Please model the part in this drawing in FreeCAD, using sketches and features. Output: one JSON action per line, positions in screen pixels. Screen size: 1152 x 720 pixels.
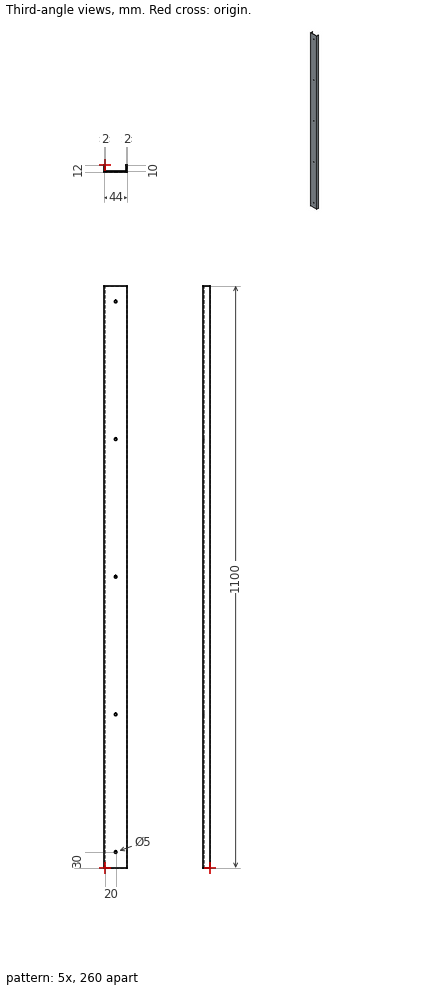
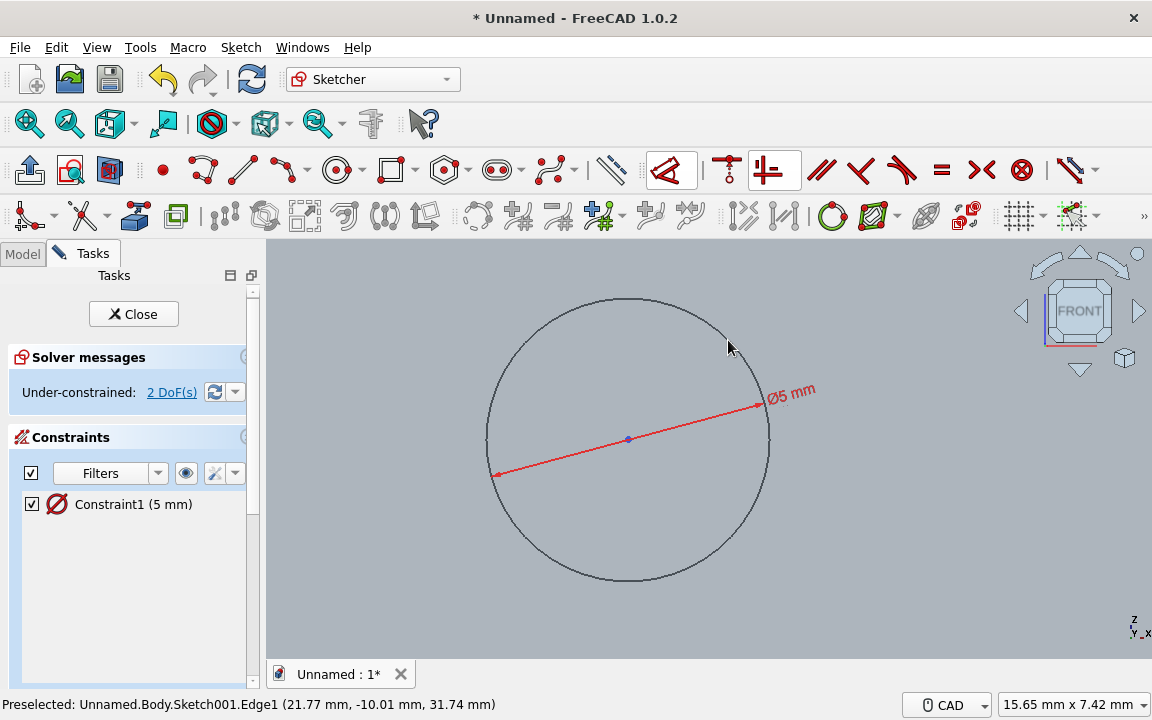
{"action": "left_click", "coordinate": [628, 440]}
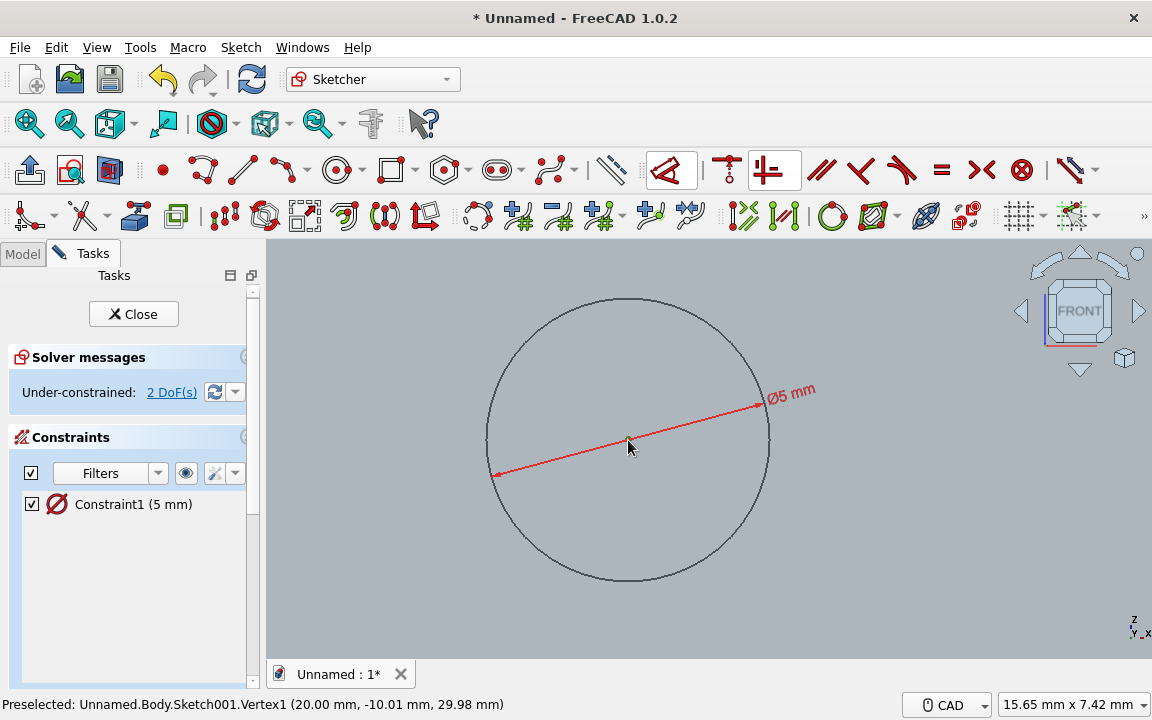
{"action": "key", "text": "l"}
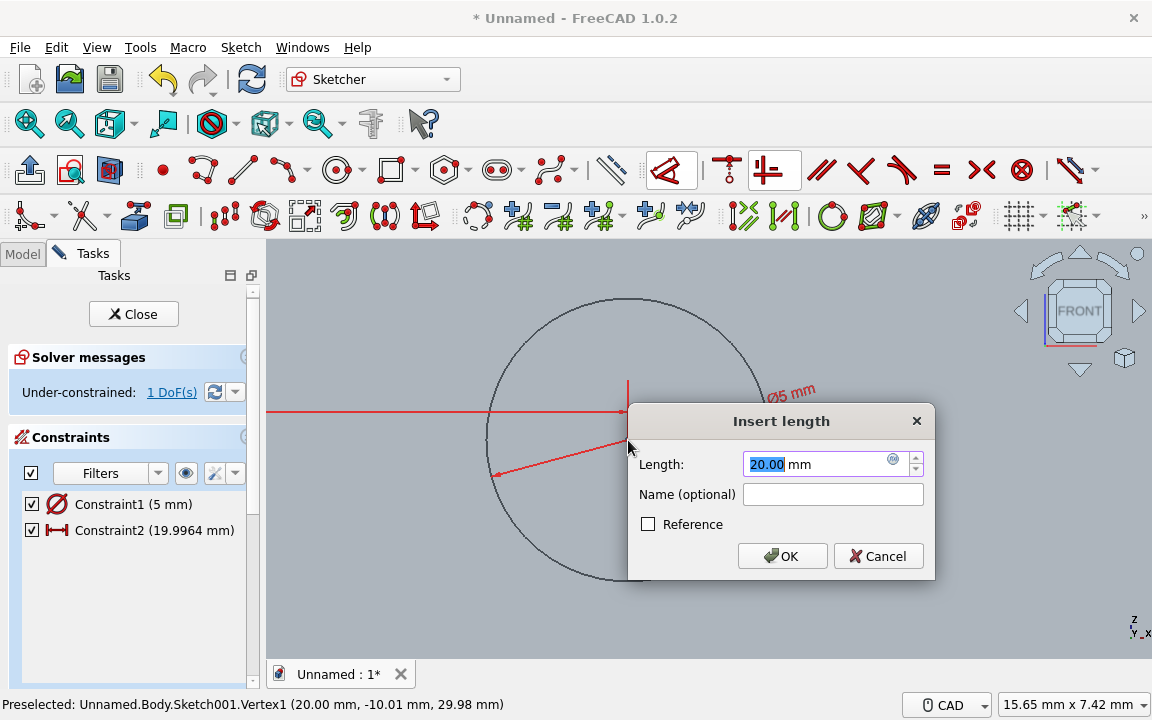
{"action": "type", "text": "20"}
{"action": "key", "text": "Return"}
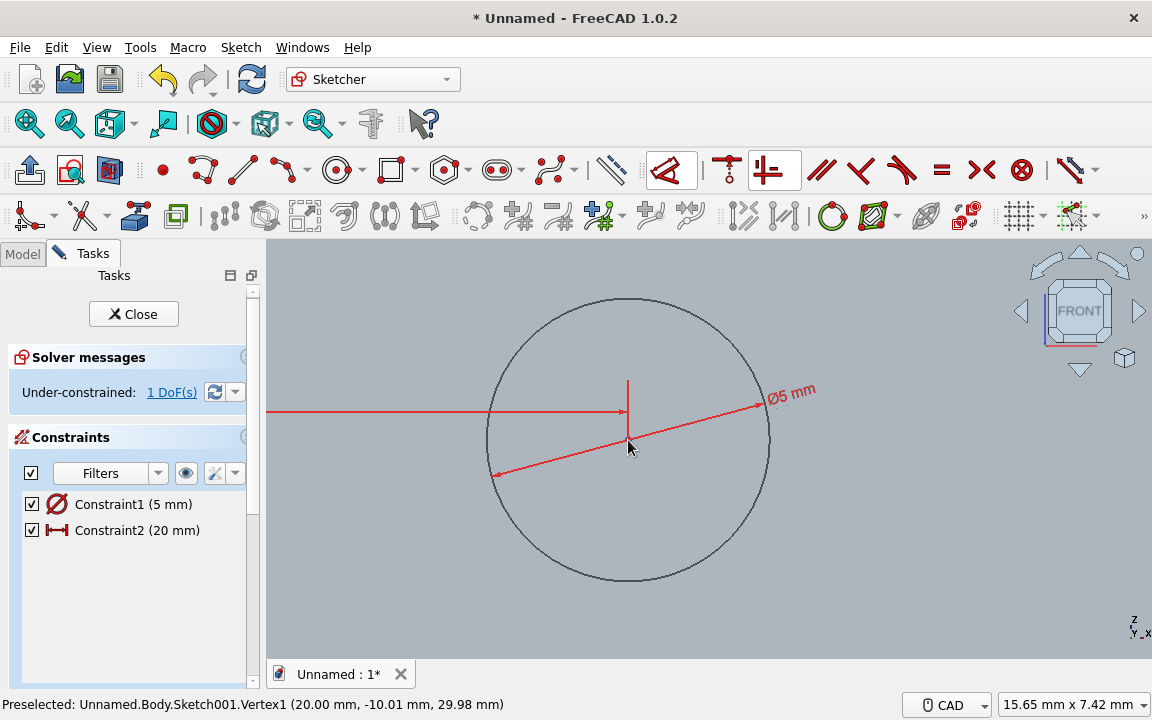
{"action": "left_click", "coordinate": [628, 440]}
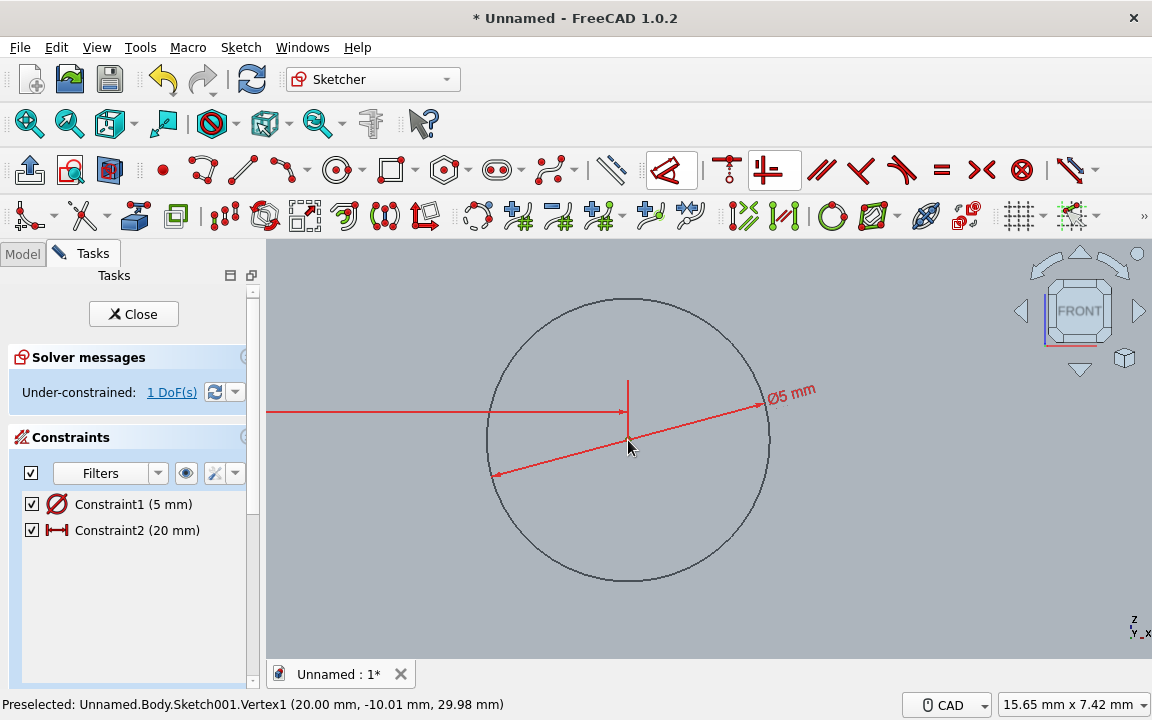
{"action": "left_click", "coordinate": [692, 170]}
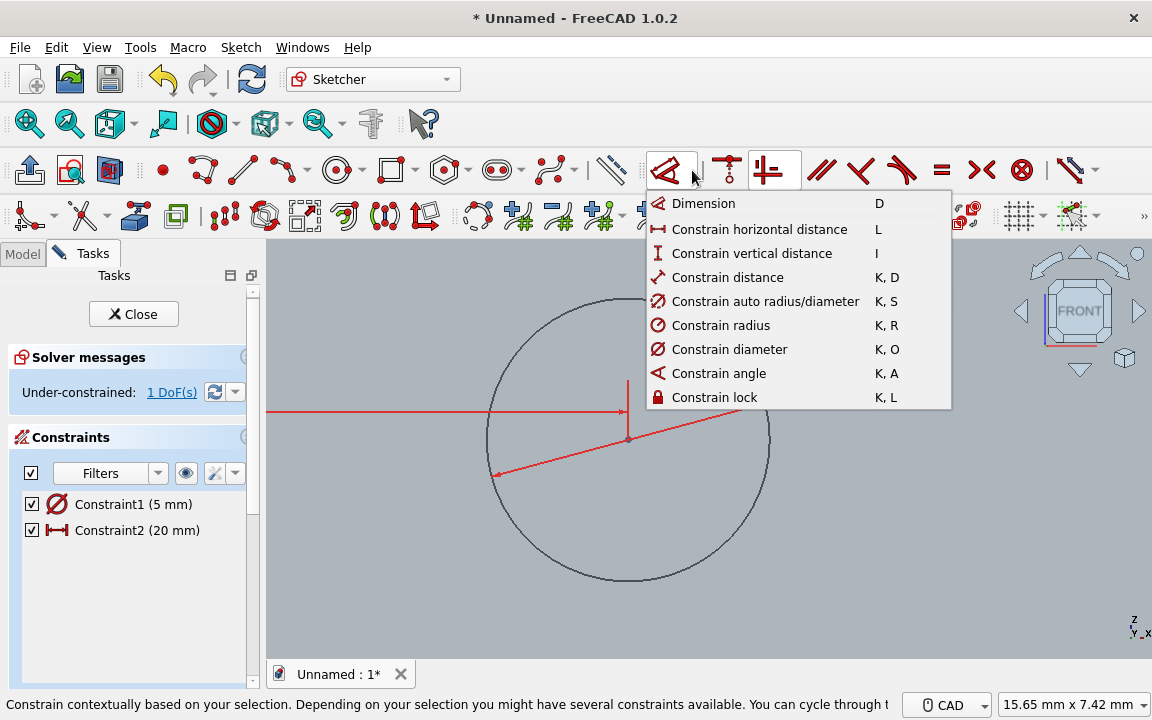
{"action": "left_click", "coordinate": [799, 253]}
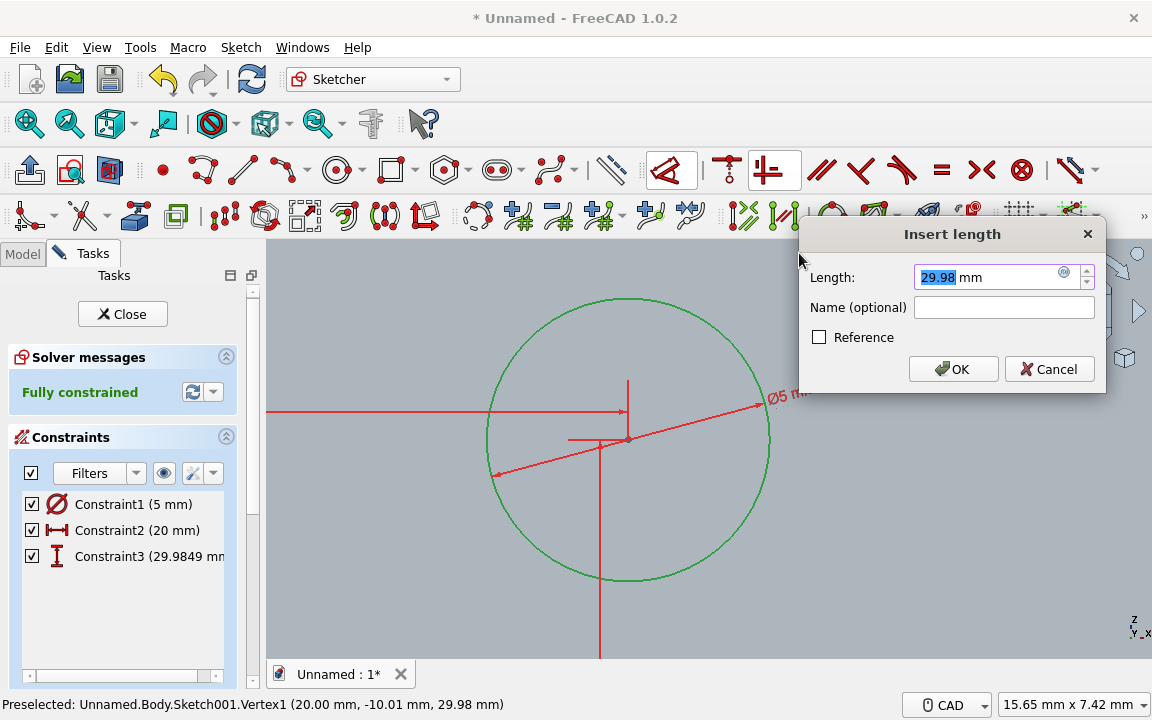
{"action": "type", "text": "30"}
{"action": "key", "text": "Return"}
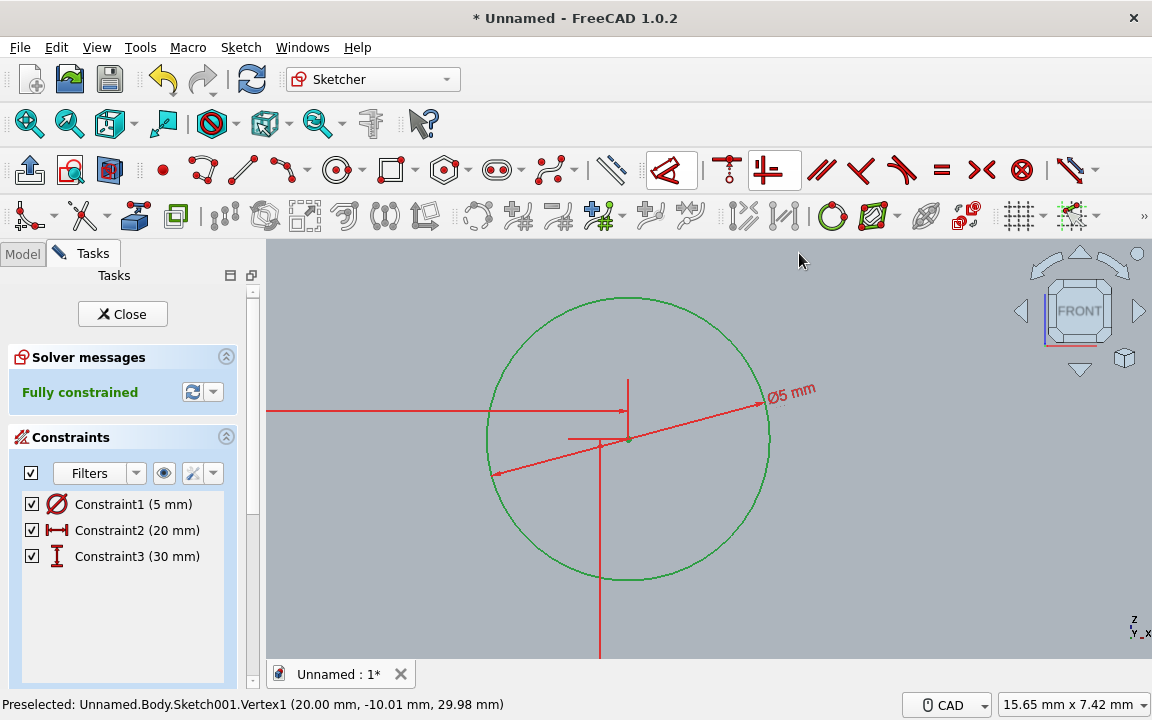
{"action": "left_click", "coordinate": [123, 314]}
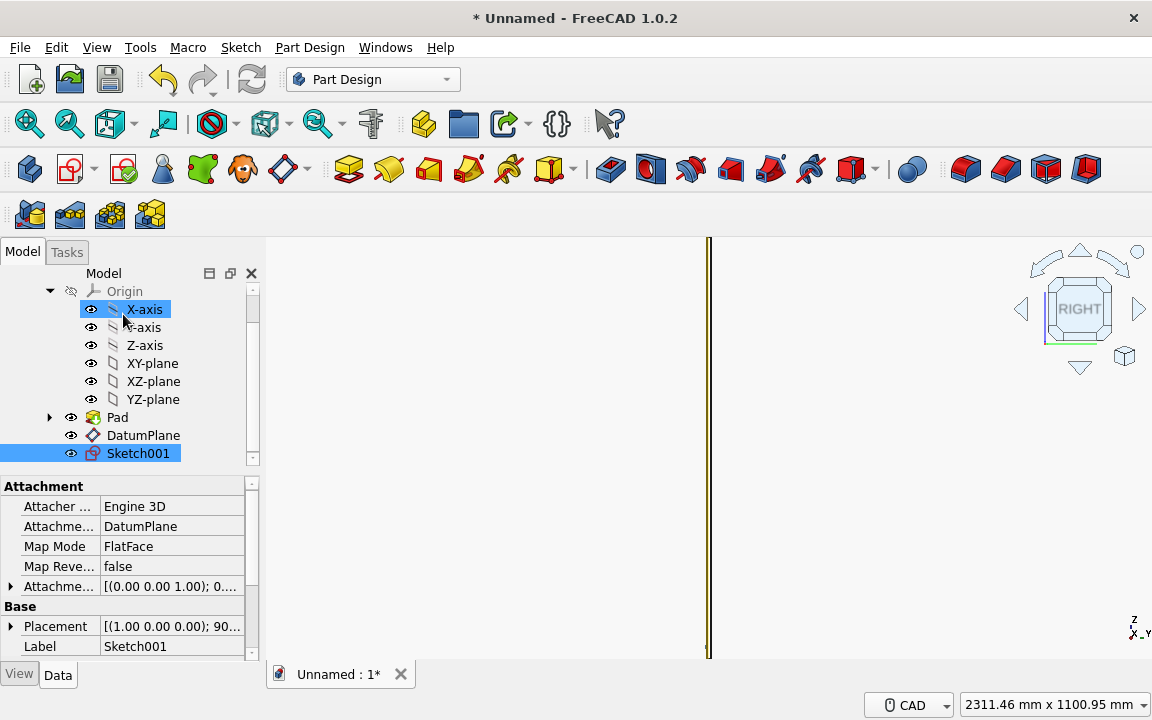
{"action": "left_click", "coordinate": [612, 170]}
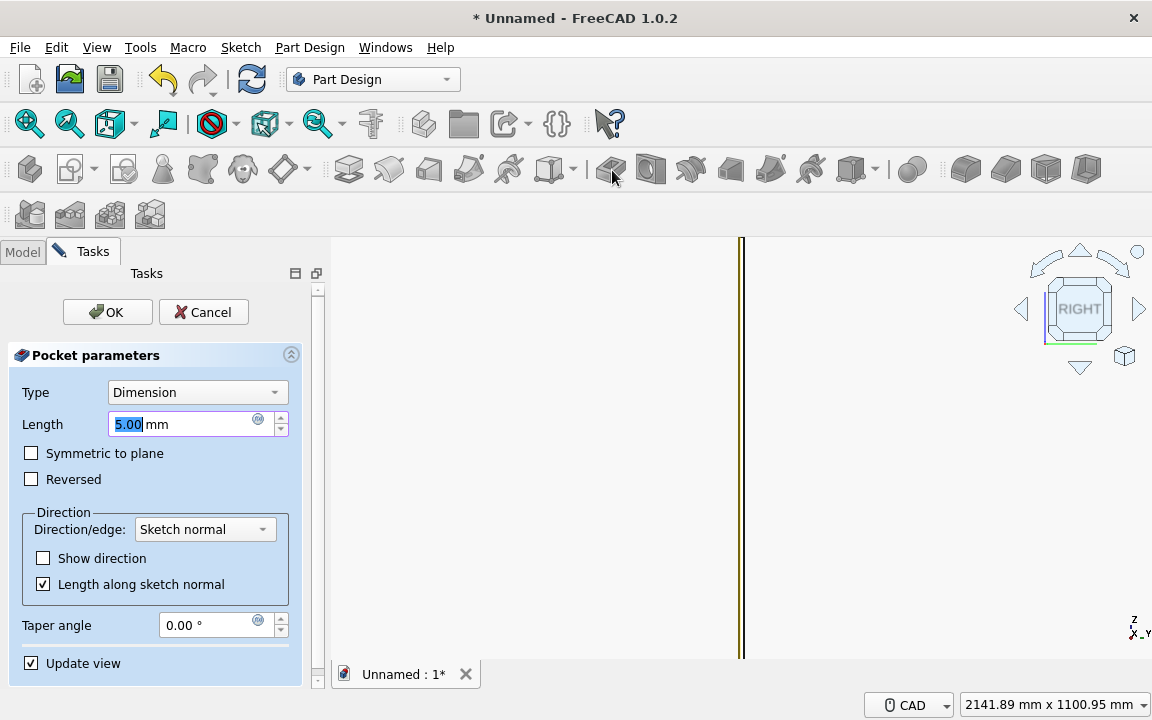
{"action": "left_click", "coordinate": [198, 392]}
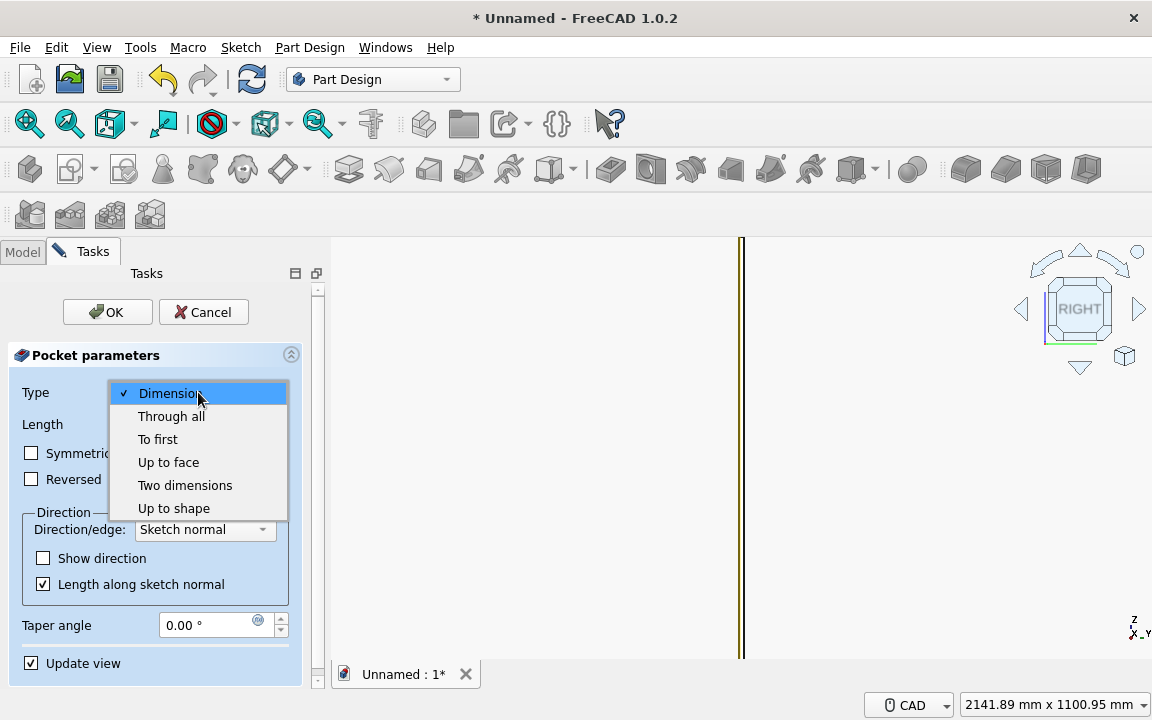
{"action": "left_click", "coordinate": [198, 416]}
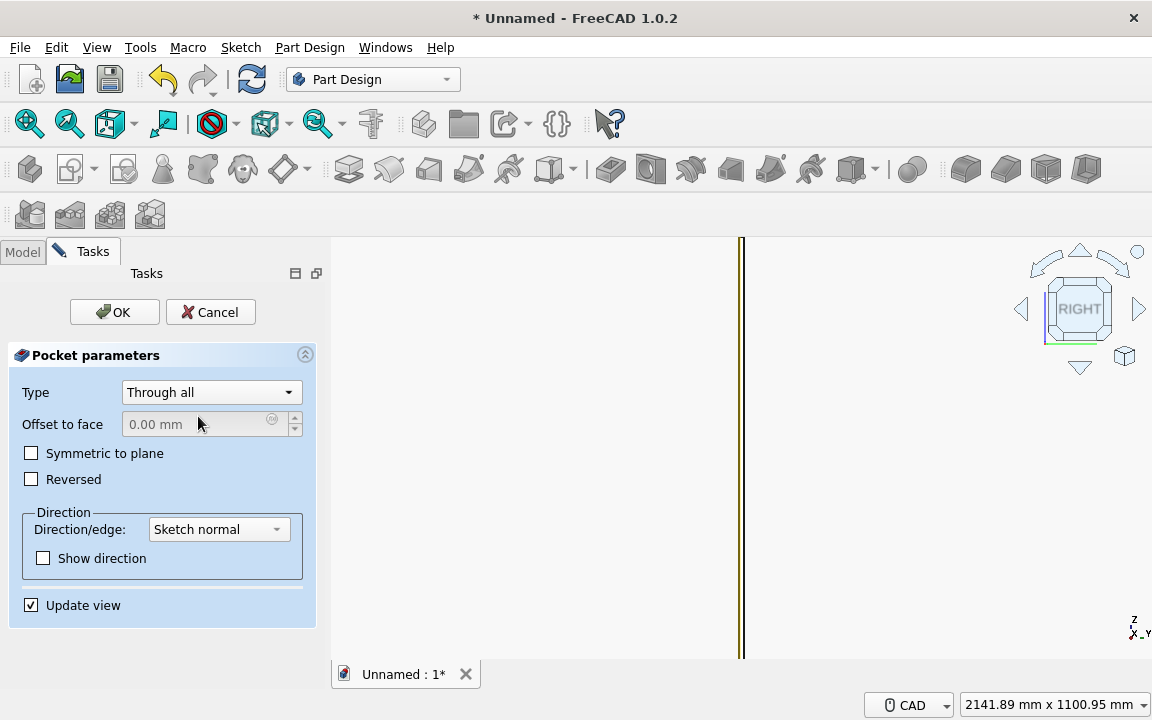
{"action": "left_click", "coordinate": [30, 479]}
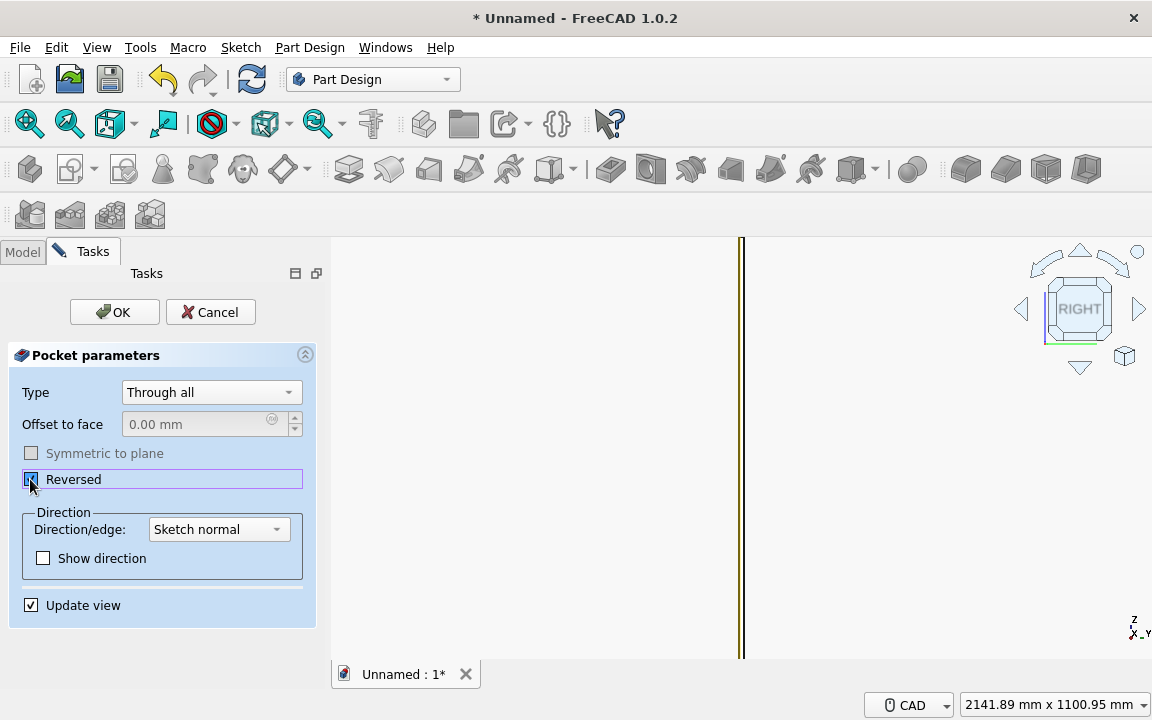
{"action": "left_click", "coordinate": [115, 312]}